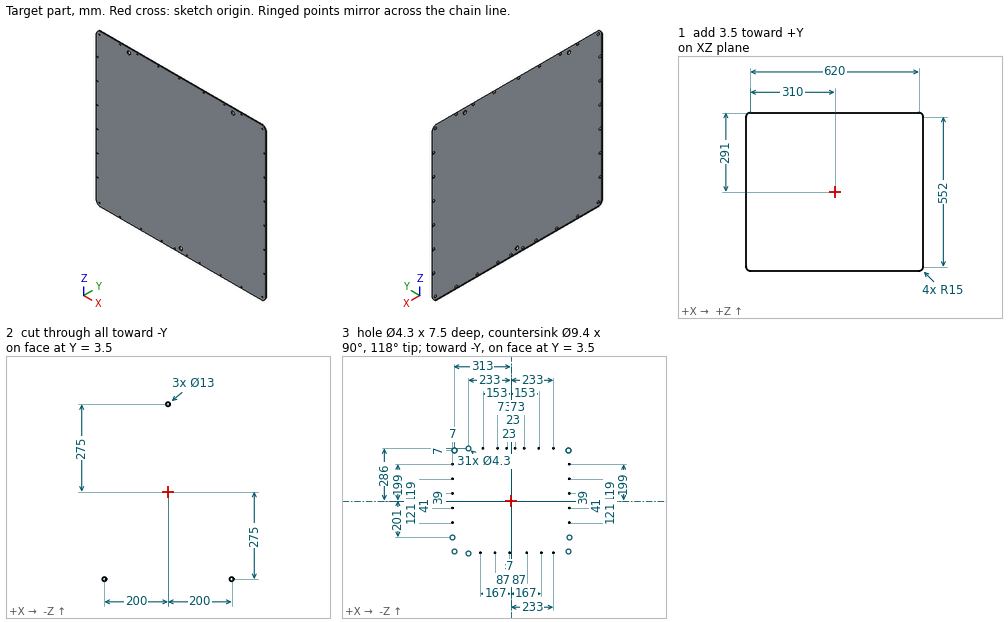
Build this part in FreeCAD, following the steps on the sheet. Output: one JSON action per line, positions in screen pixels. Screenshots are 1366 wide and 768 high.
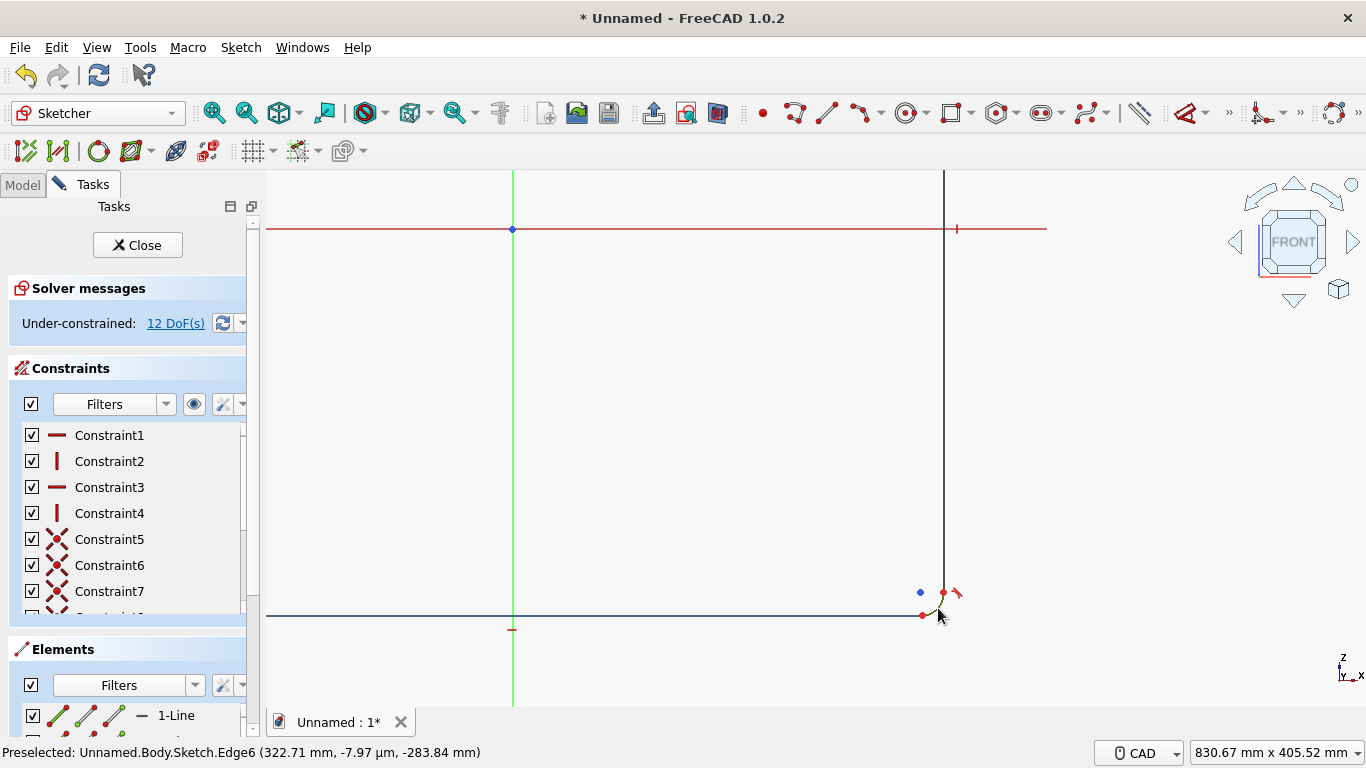
{"action": "key", "text": "t"}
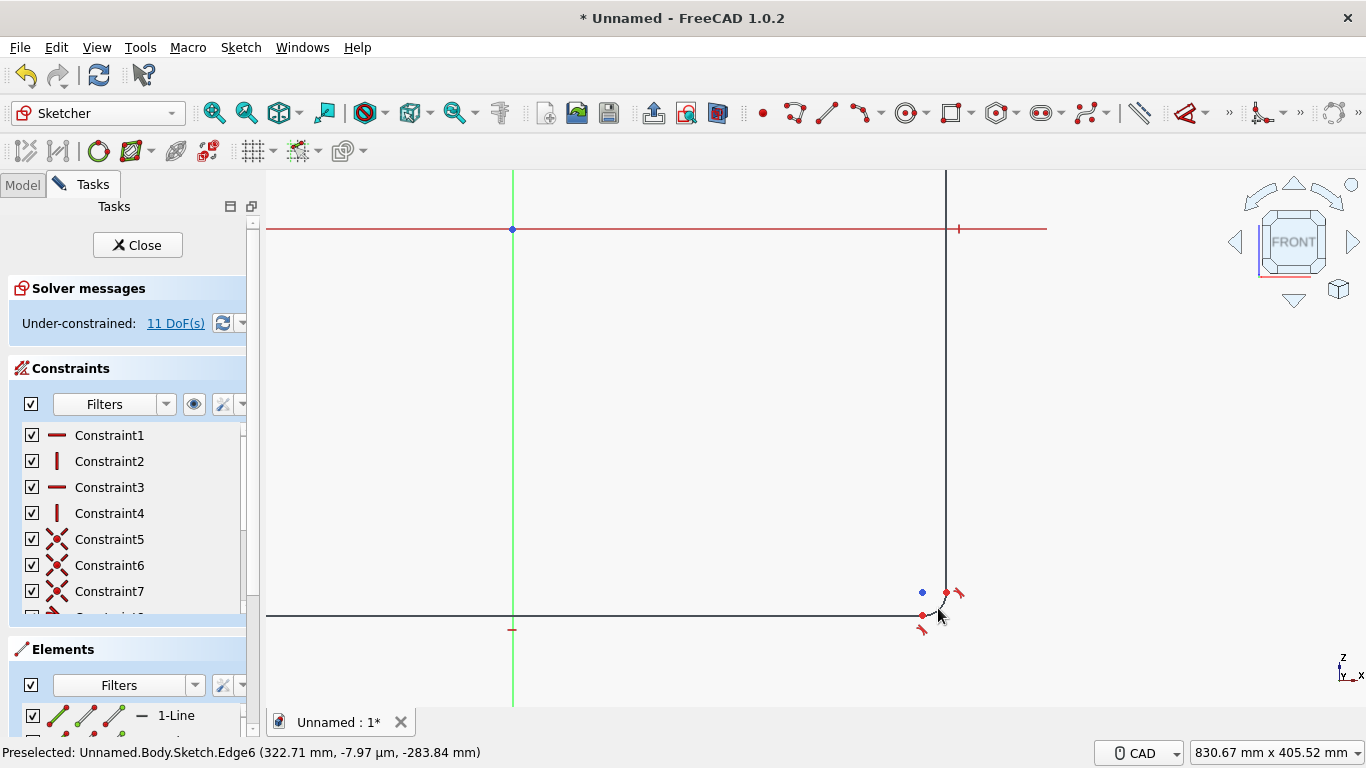
{"action": "left_click", "coordinate": [677, 616]}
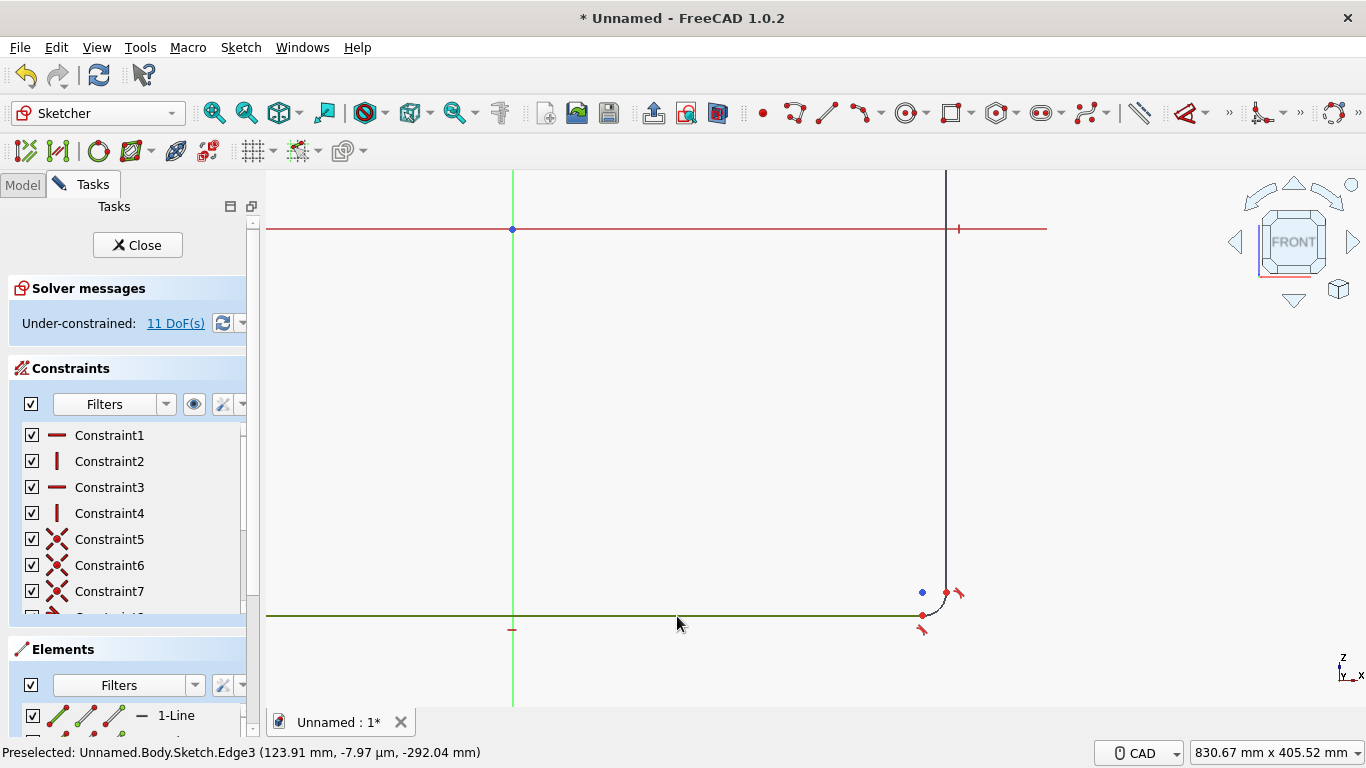
{"action": "scroll", "coordinate": [939, 609], "scroll_direction": "down", "scroll_amount": 4}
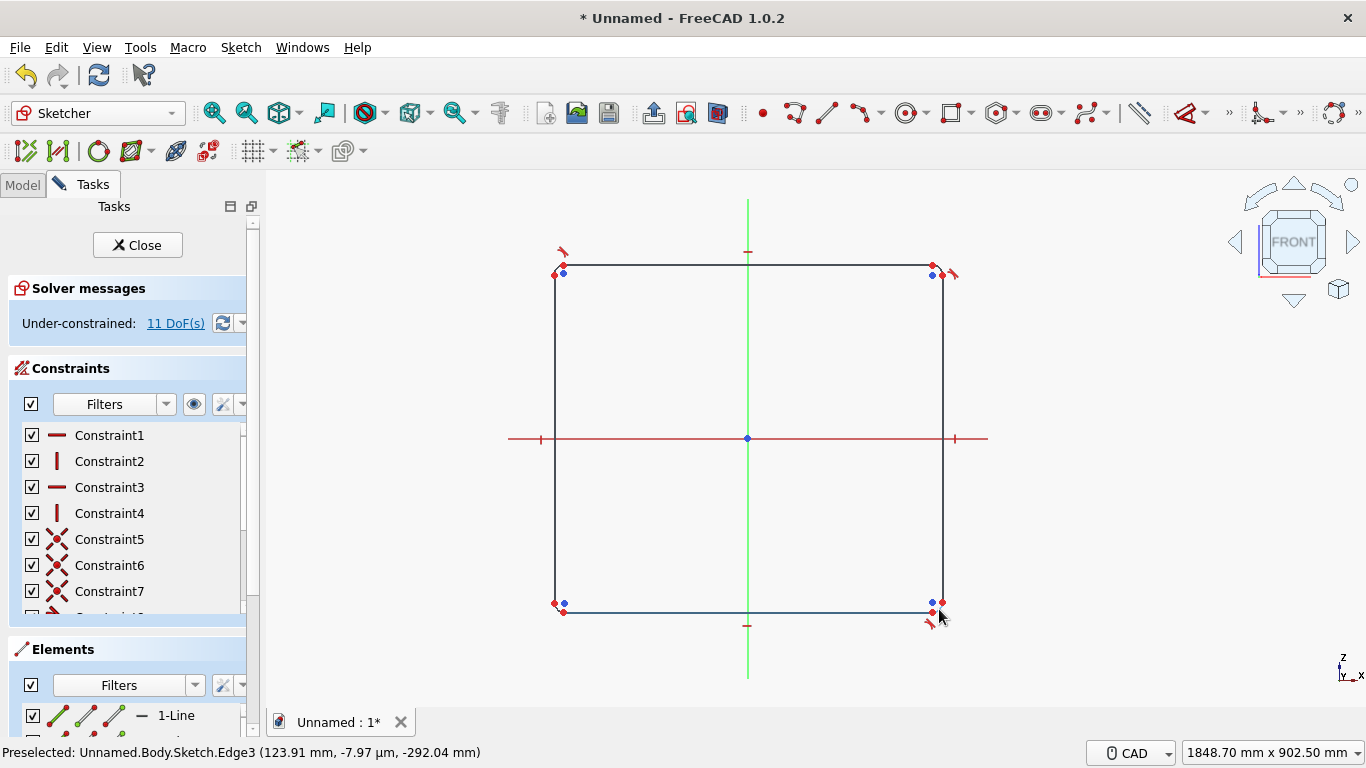
{"action": "scroll", "coordinate": [558, 610], "scroll_direction": "up", "scroll_amount": 4}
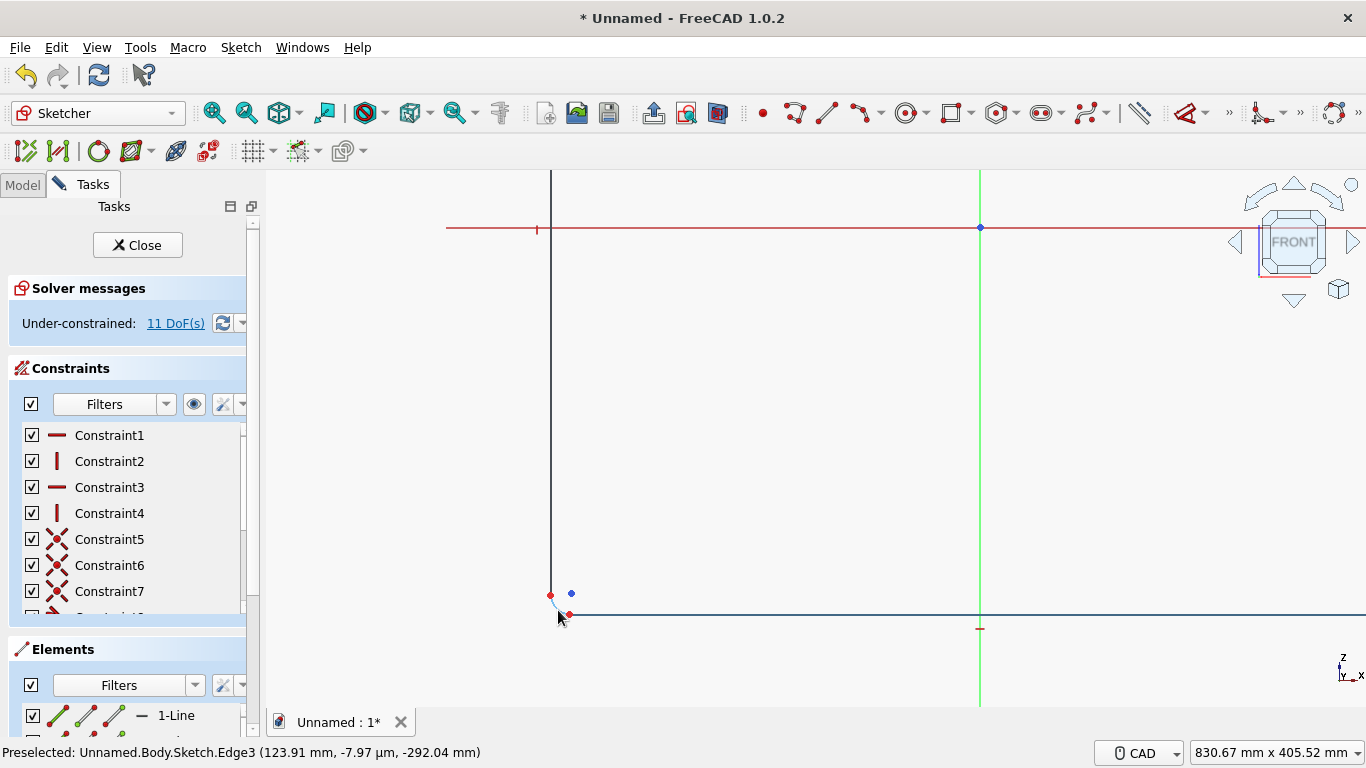
{"action": "left_click", "coordinate": [557, 609]}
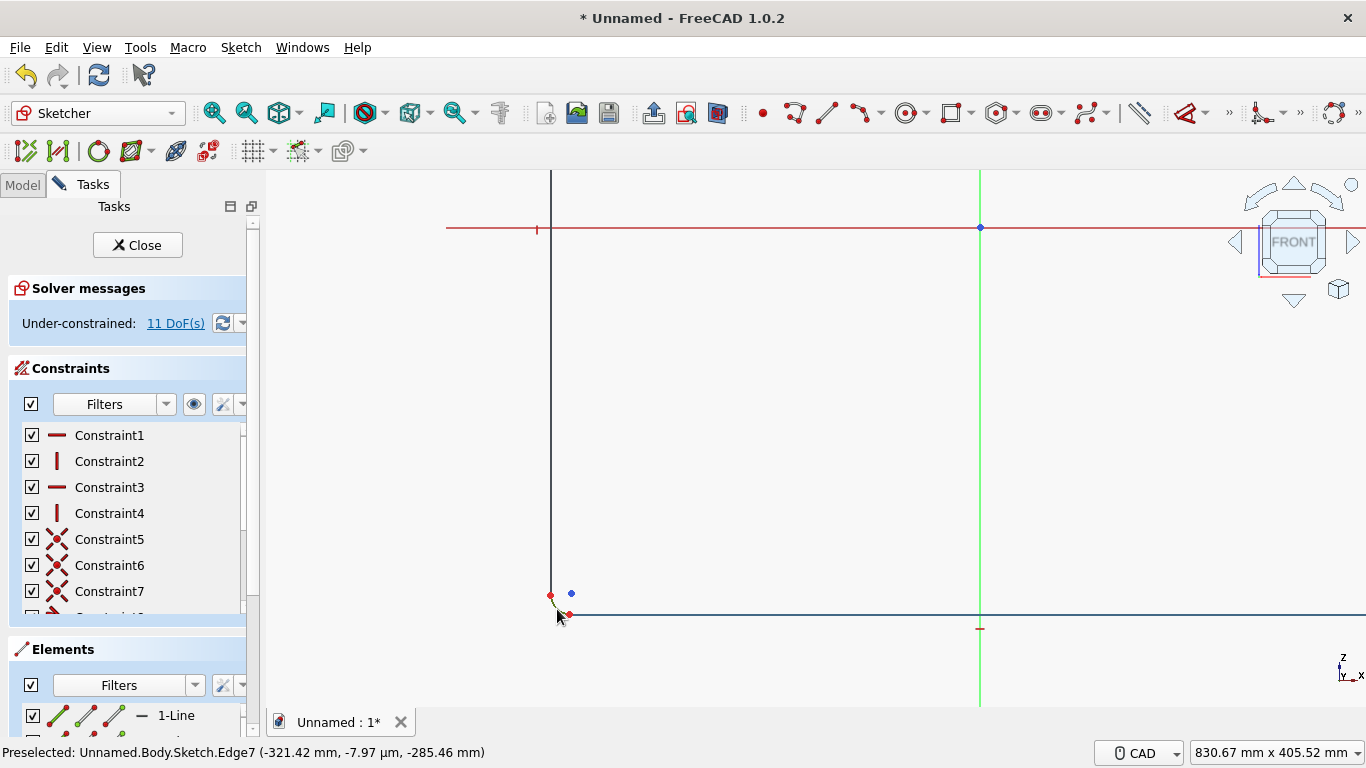
{"action": "key", "text": "t"}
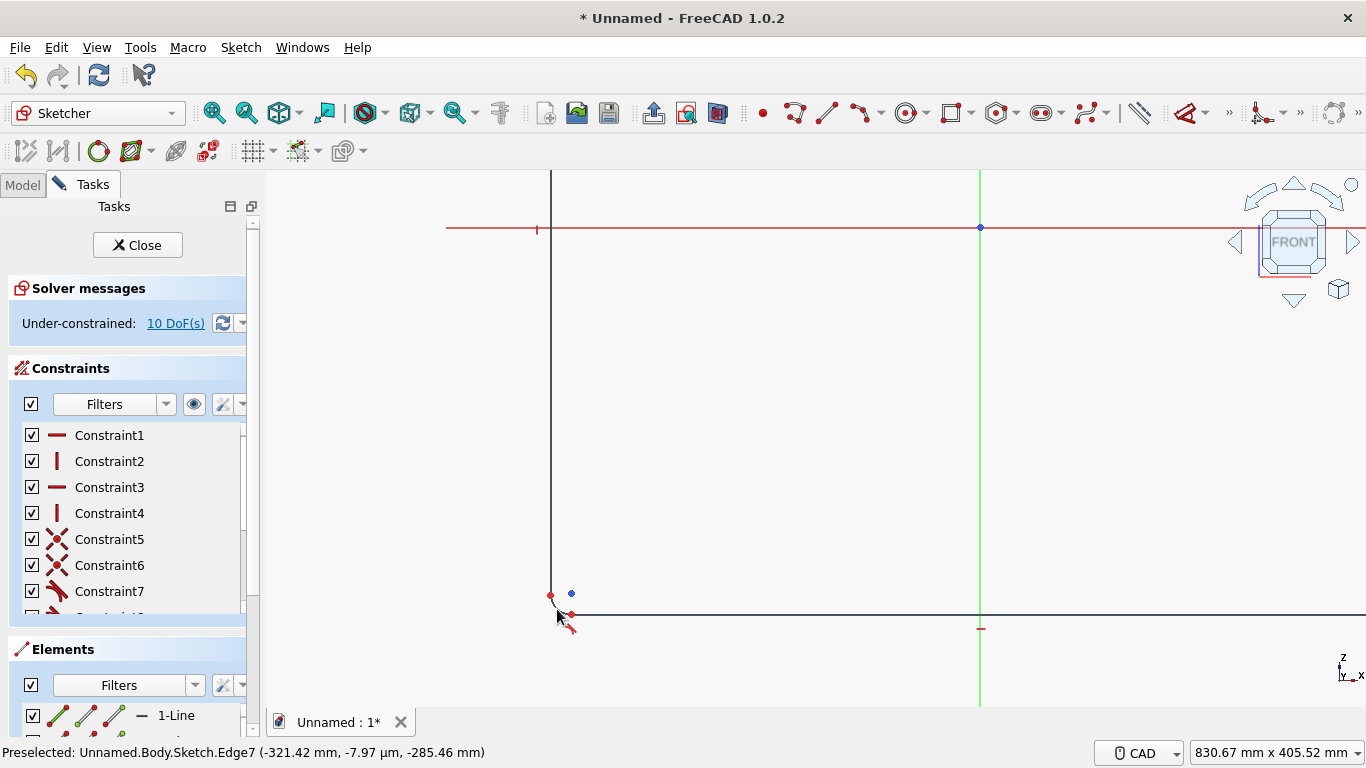
{"action": "left_click", "coordinate": [551, 376]}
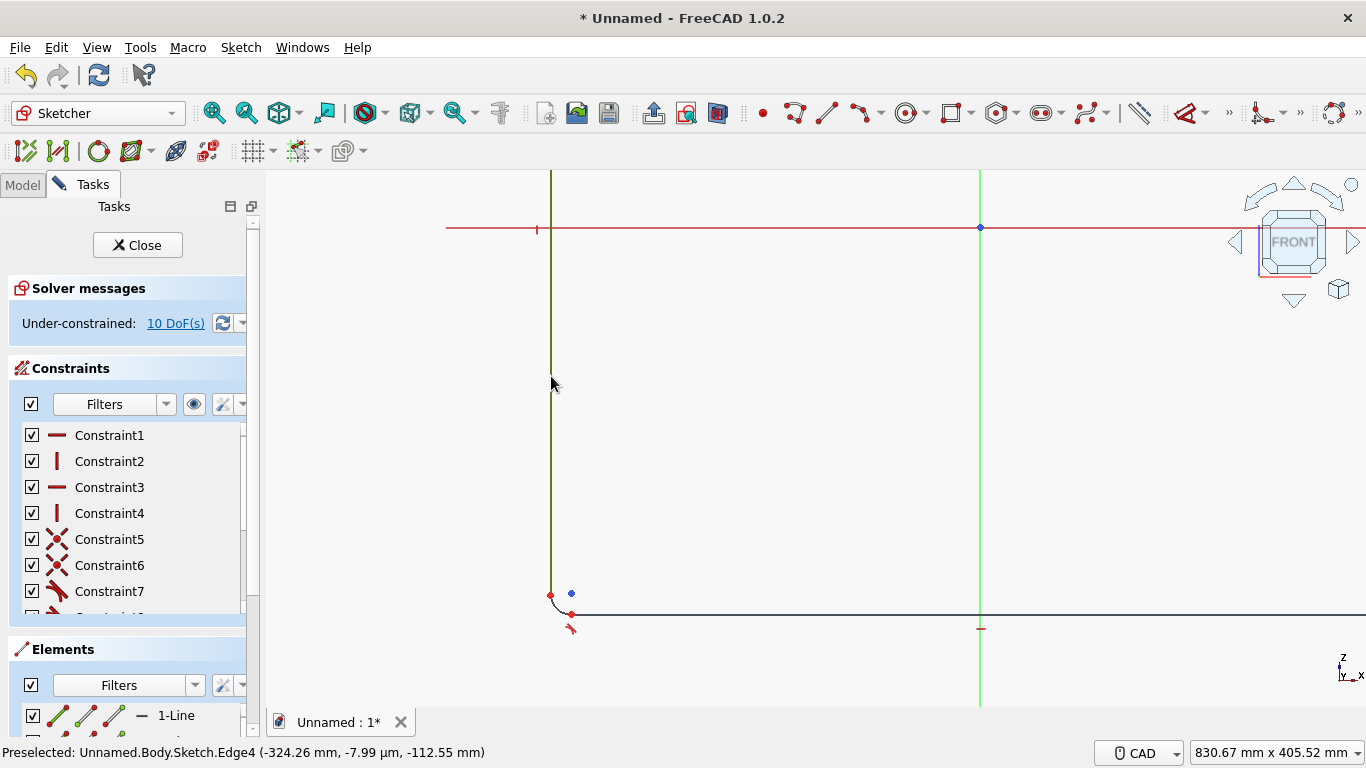
{"action": "scroll", "coordinate": [554, 604], "scroll_direction": "up", "scroll_amount": 3}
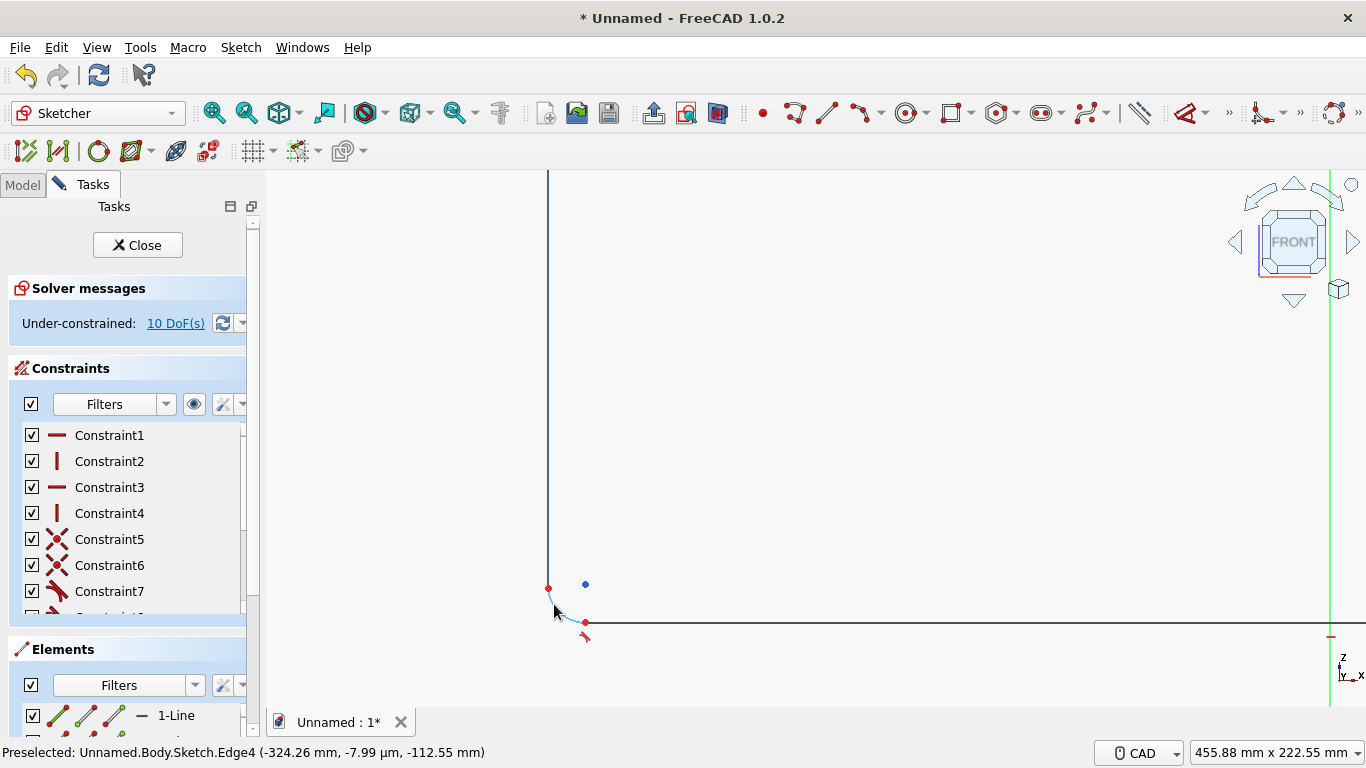
{"action": "left_click", "coordinate": [553, 604]}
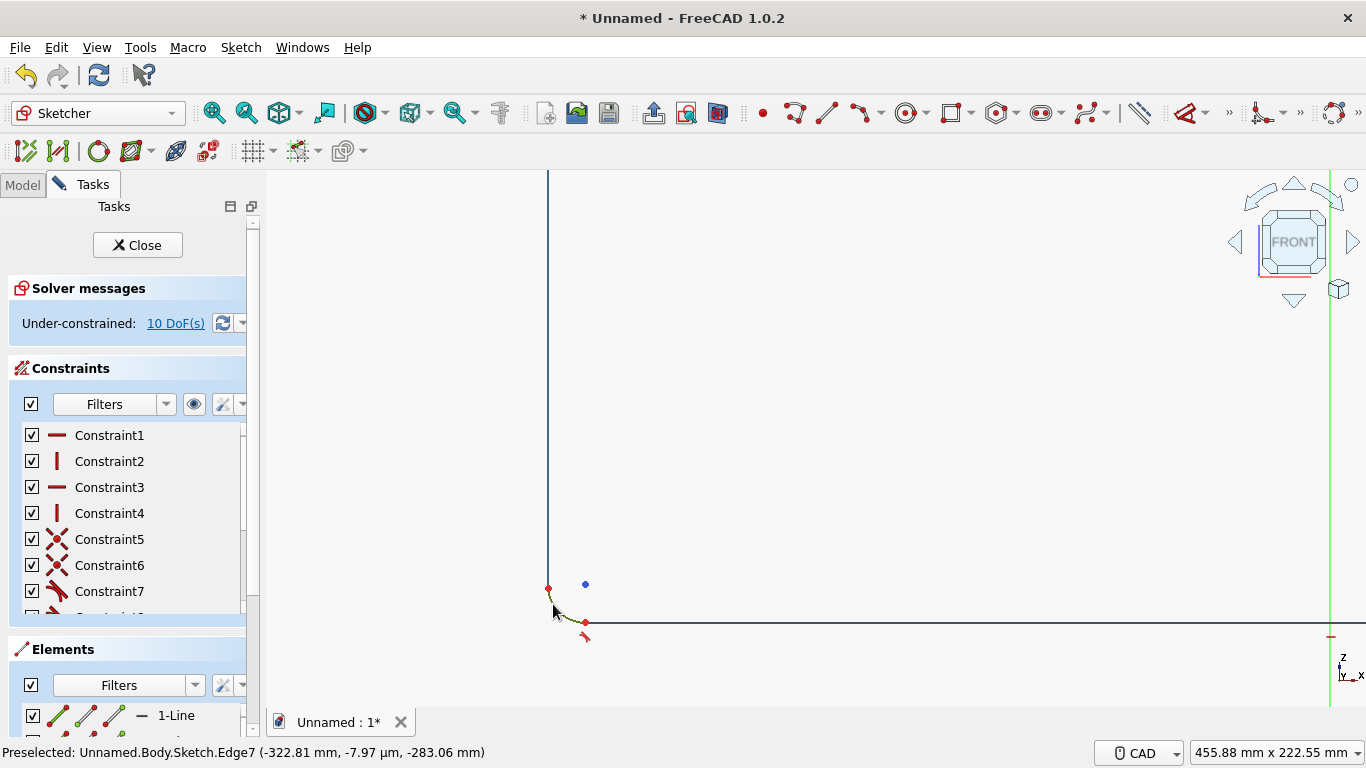
{"action": "key", "text": "t"}